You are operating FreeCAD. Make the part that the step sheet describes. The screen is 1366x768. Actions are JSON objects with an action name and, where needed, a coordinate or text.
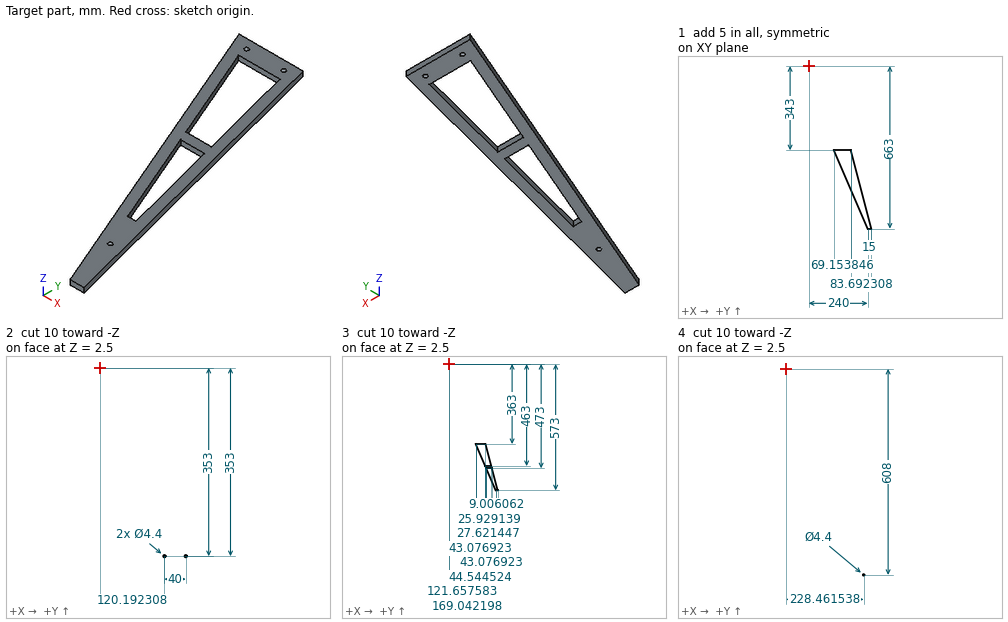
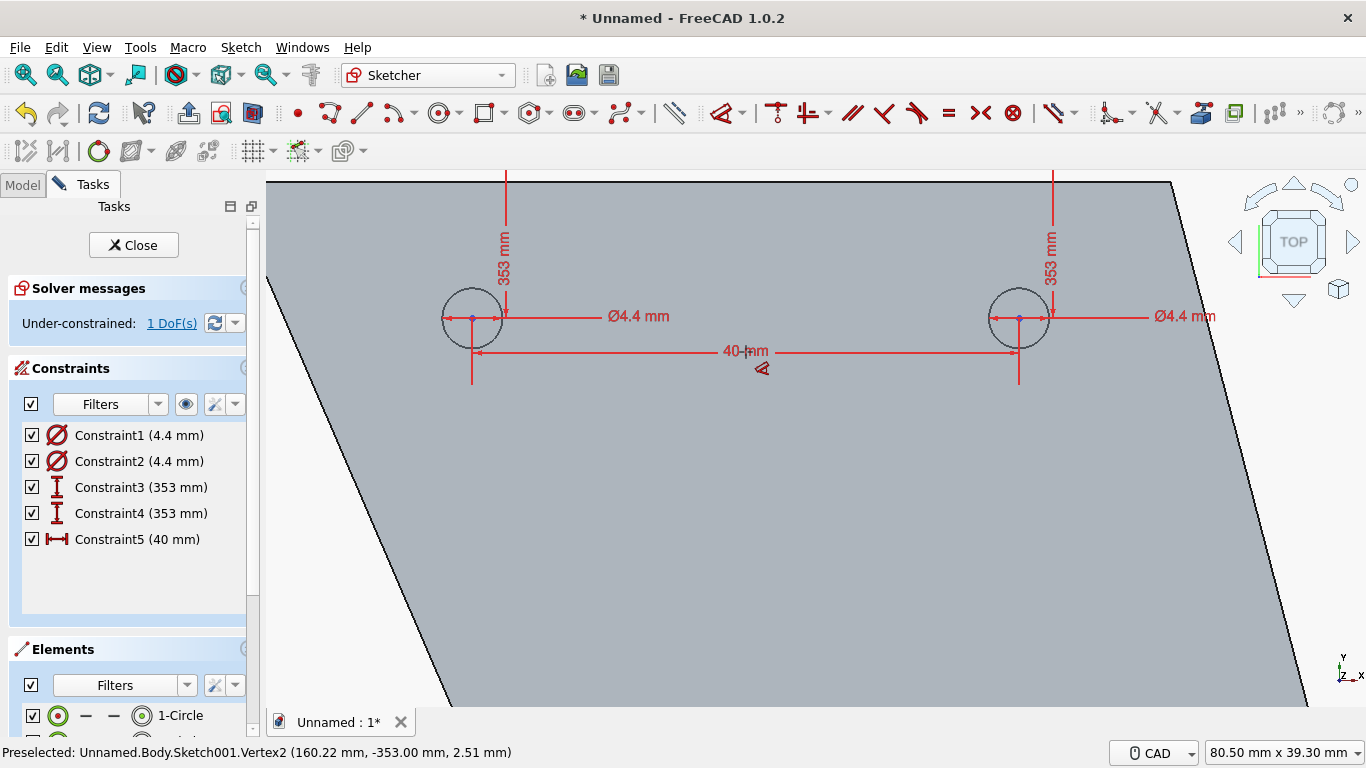
{"action": "left_click", "coordinate": [472, 318]}
{"action": "left_click", "coordinate": [383, 352]}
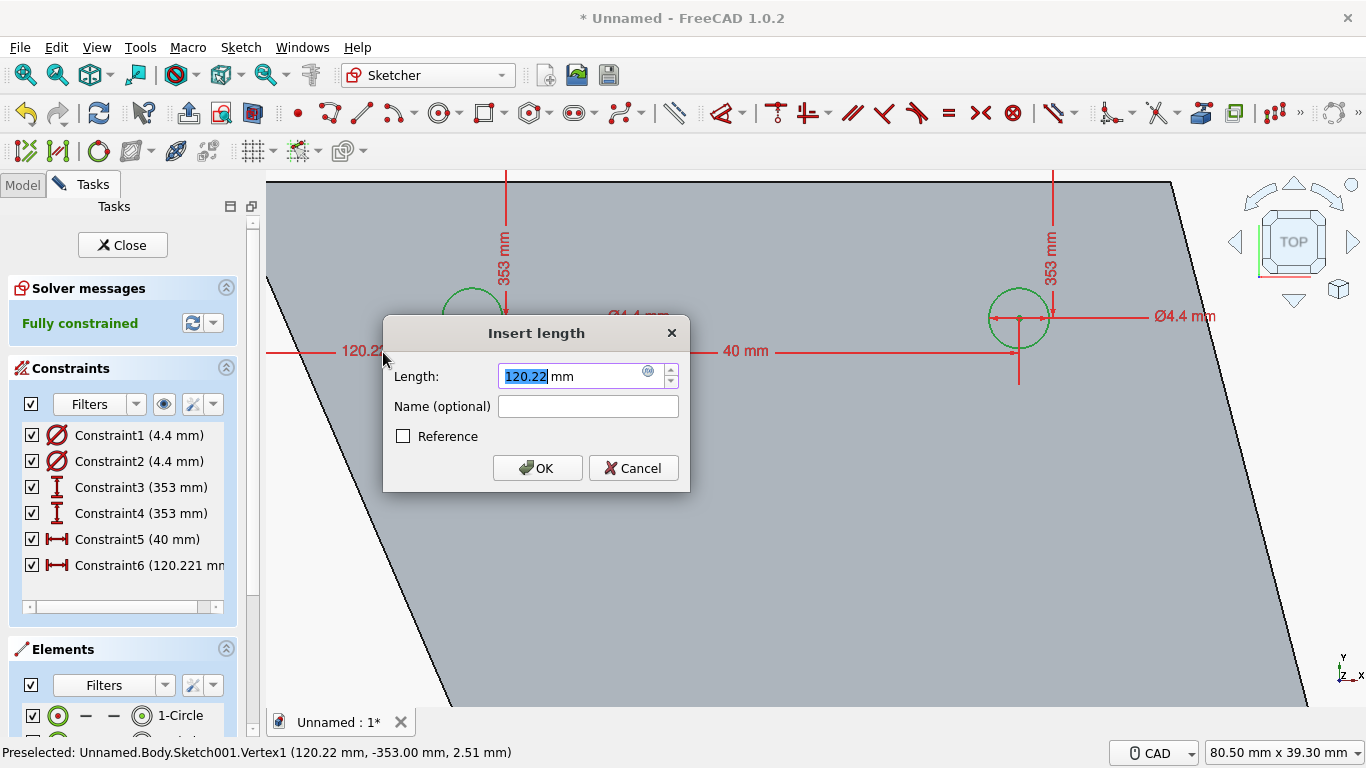
{"action": "type", "text": "120.192308"}
{"action": "key", "text": "Return"}
{"action": "key", "text": "Escape"}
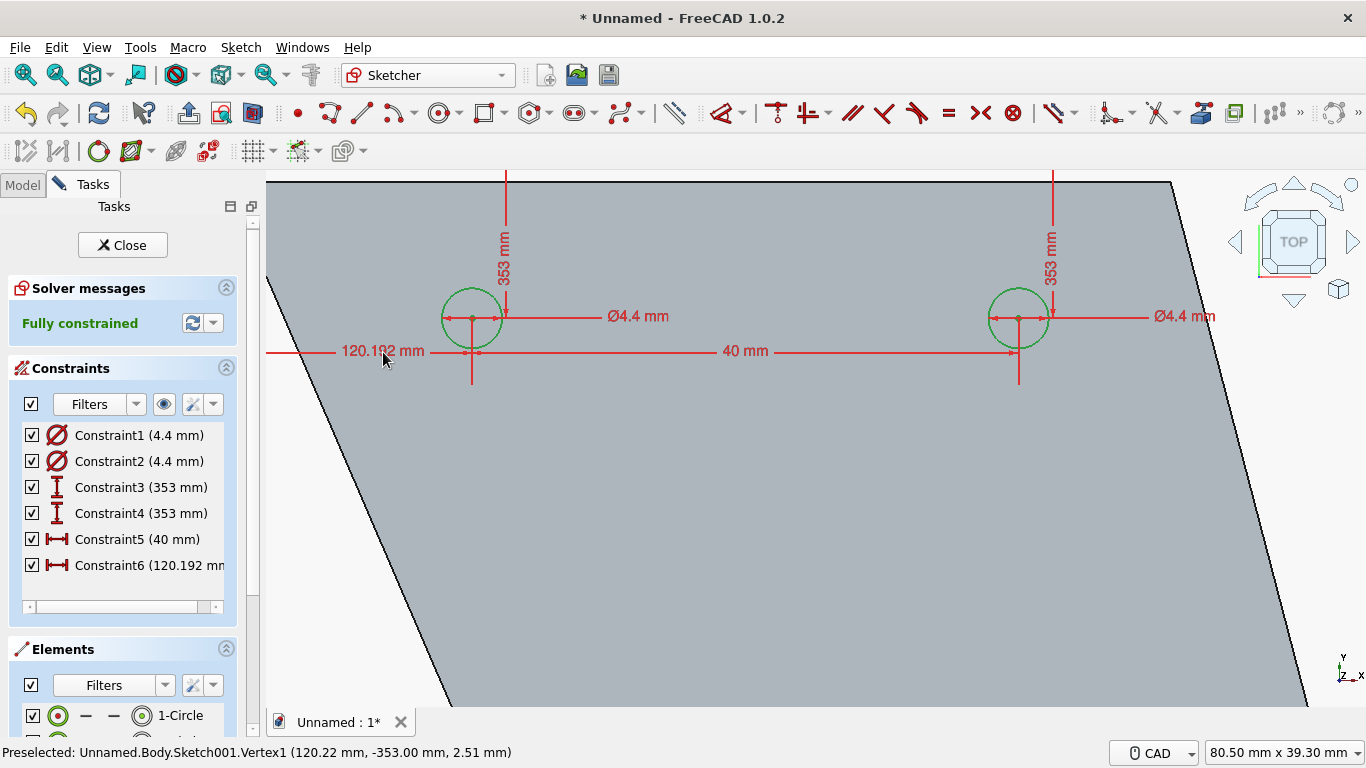
{"action": "left_click", "coordinate": [123, 245]}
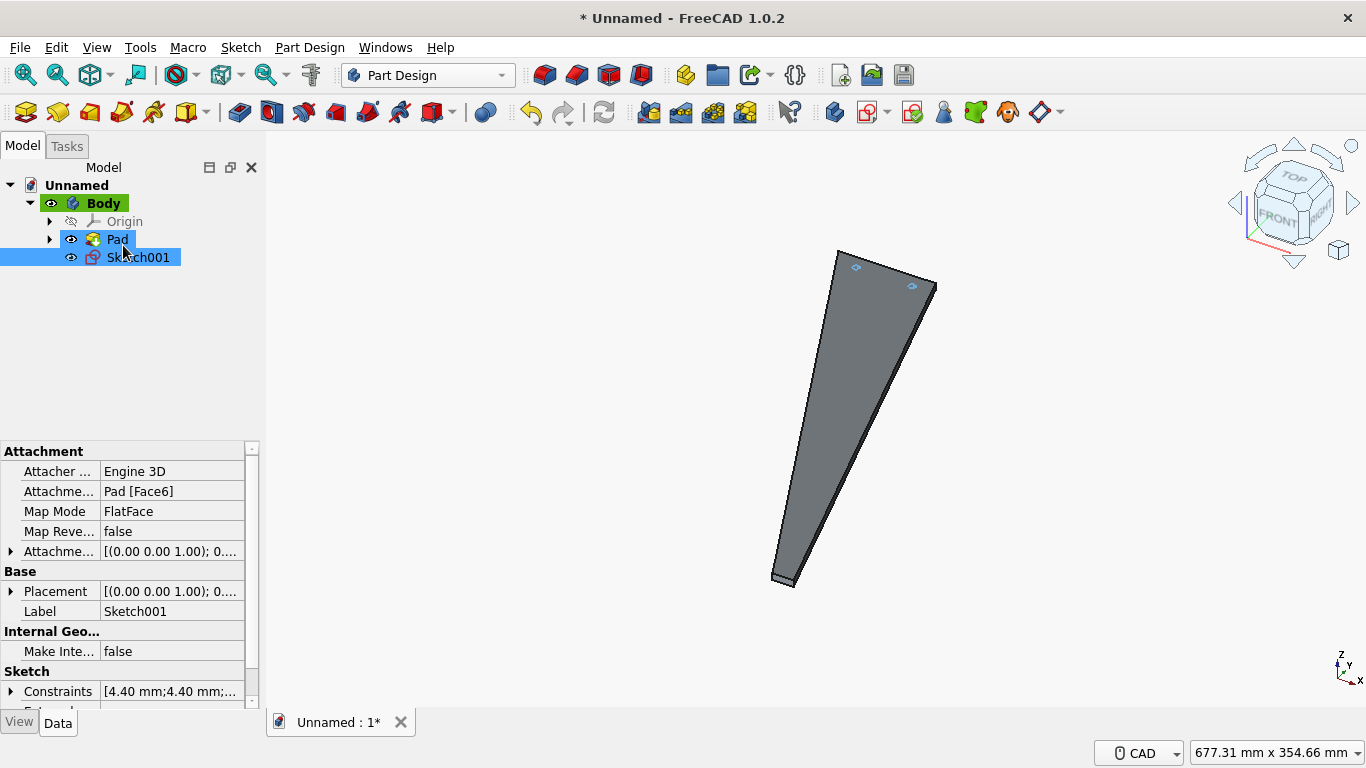
{"action": "left_click", "coordinate": [240, 112]}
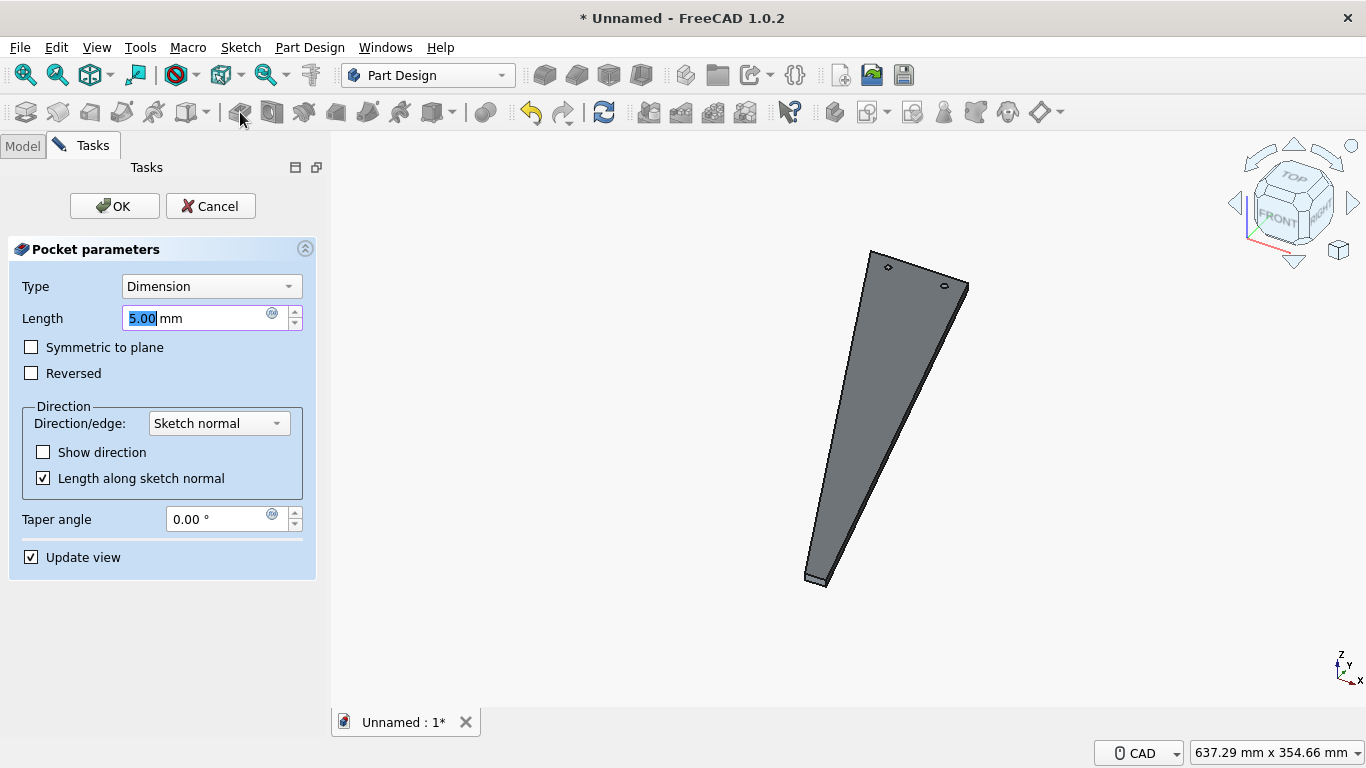
{"action": "type", "text": "10"}
{"action": "key", "text": "Tab"}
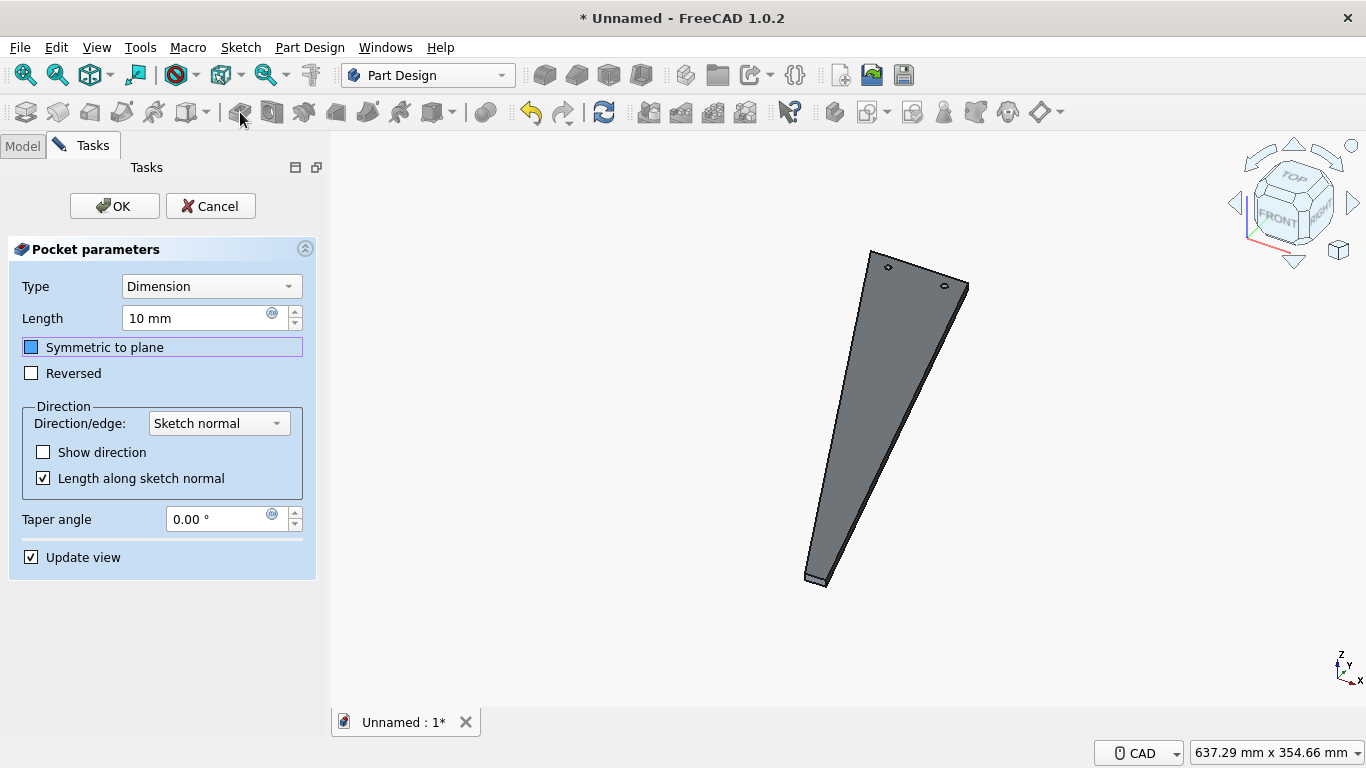
{"action": "left_click", "coordinate": [115, 206]}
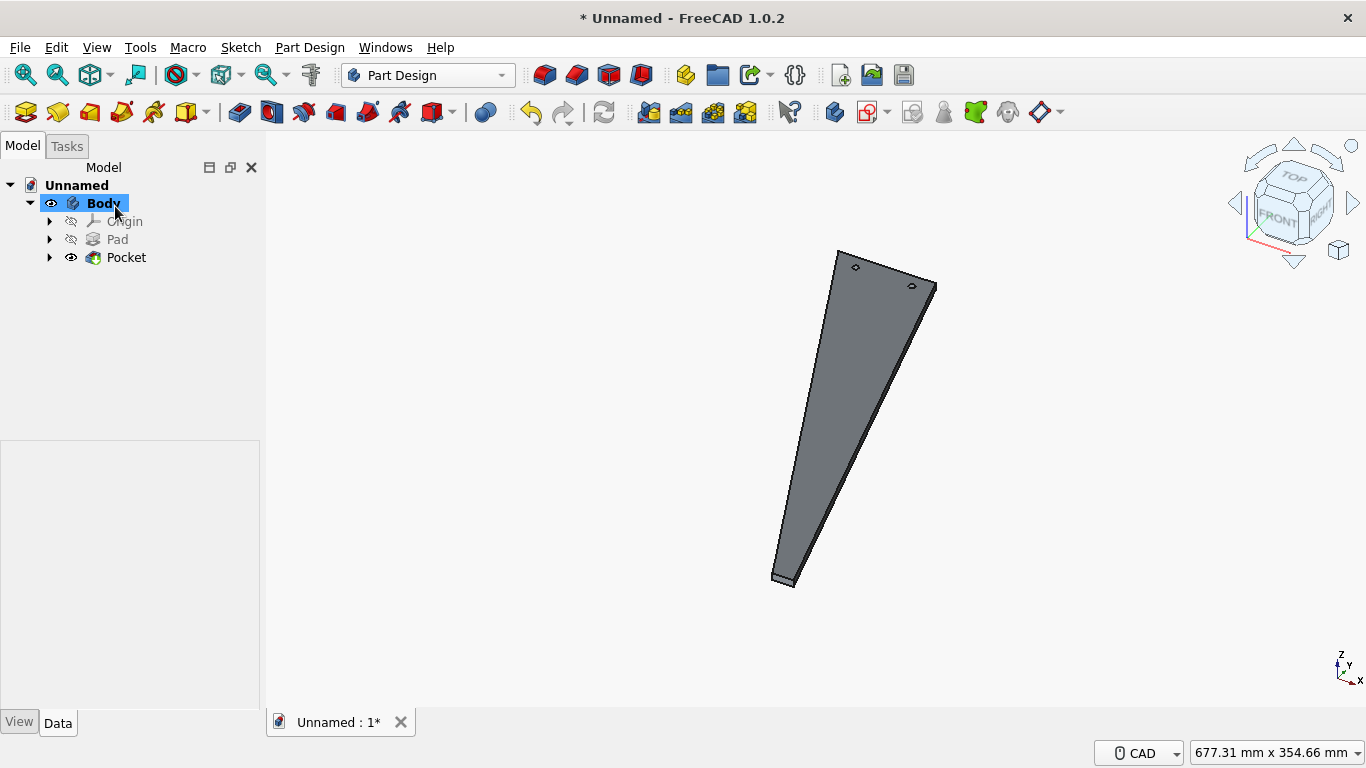
{"action": "left_click", "coordinate": [860, 331]}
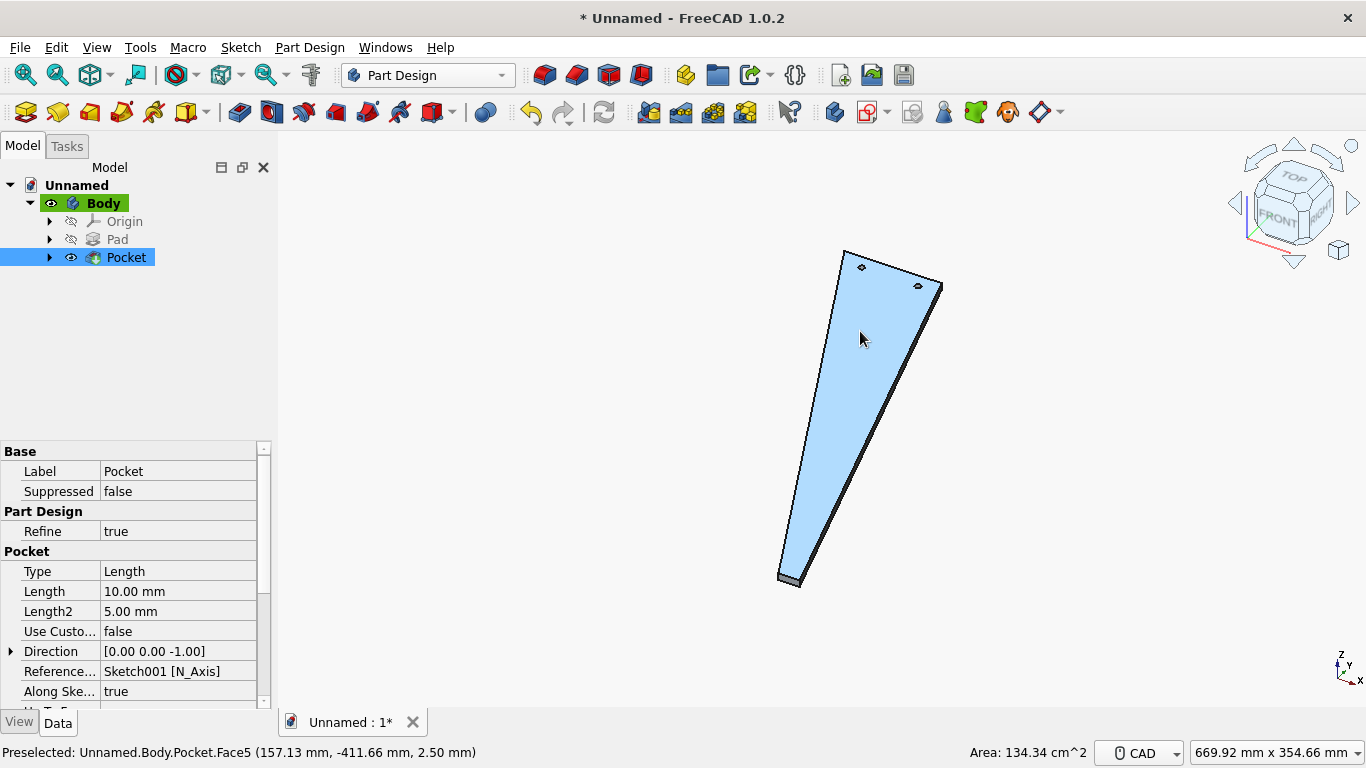
{"action": "left_click", "coordinate": [868, 112]}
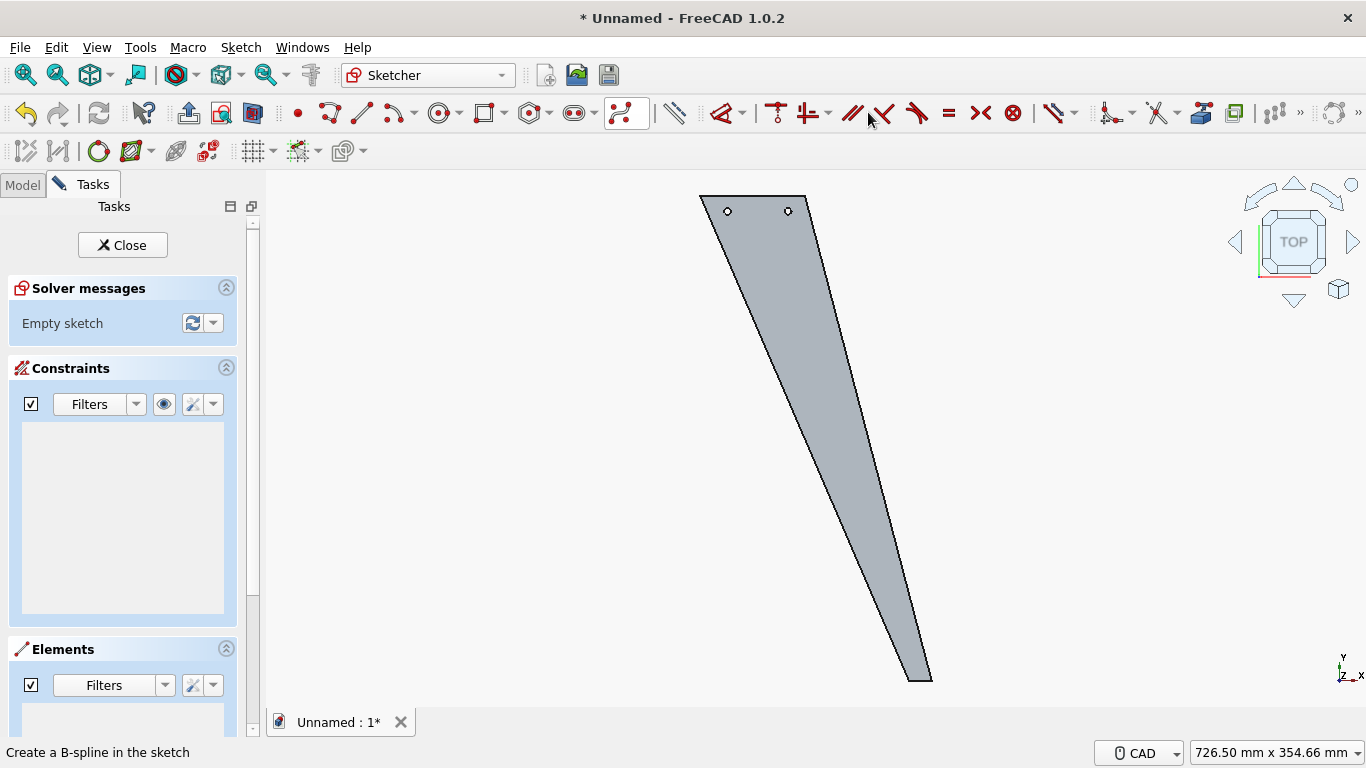
{"action": "key", "text": "g m"}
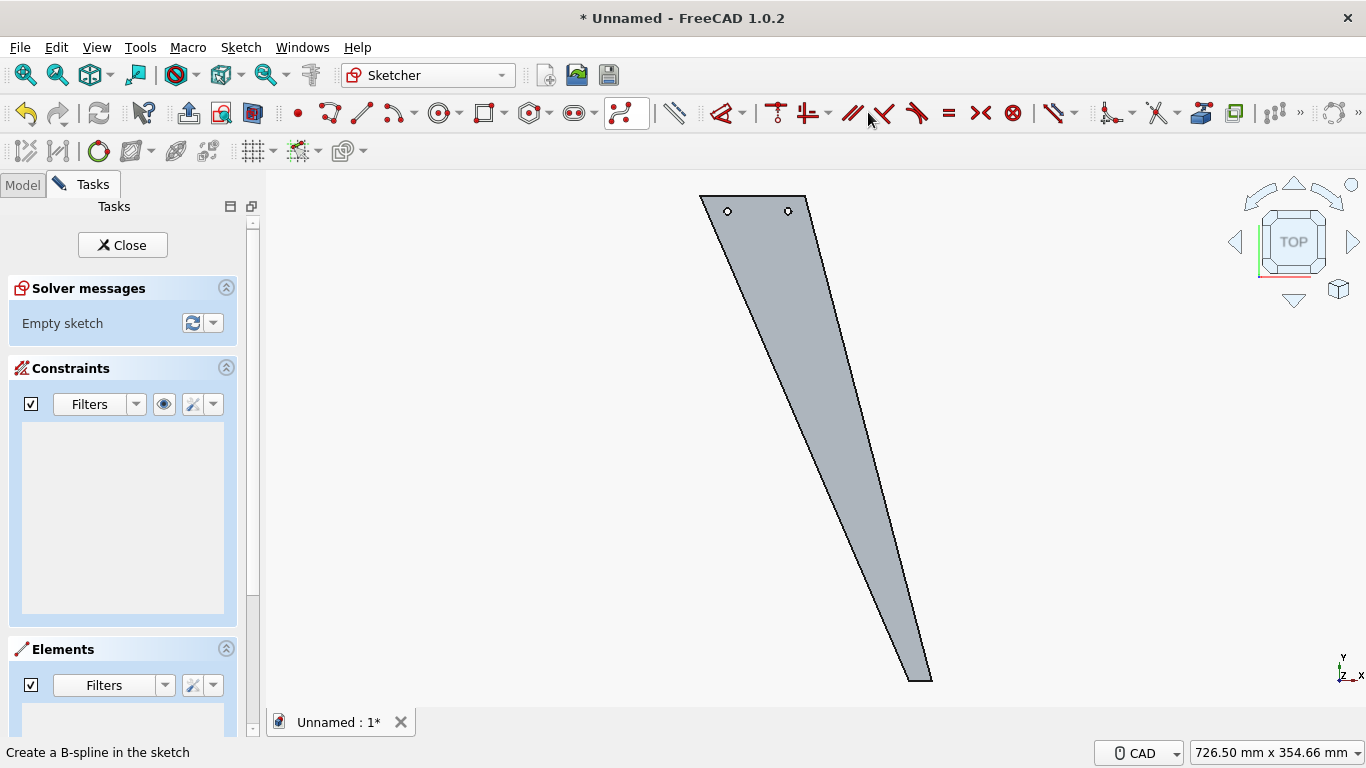
{"action": "left_click", "coordinate": [730, 227]}
{"action": "left_click", "coordinate": [795, 378]}
{"action": "left_click", "coordinate": [837, 378]}
{"action": "left_click", "coordinate": [797, 227]}
{"action": "left_click", "coordinate": [730, 228]}